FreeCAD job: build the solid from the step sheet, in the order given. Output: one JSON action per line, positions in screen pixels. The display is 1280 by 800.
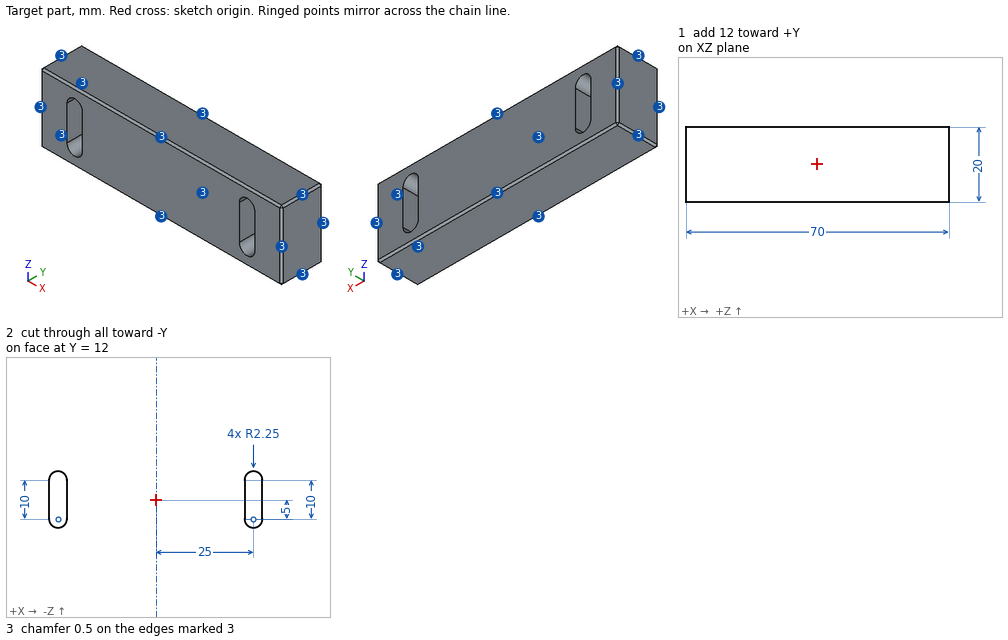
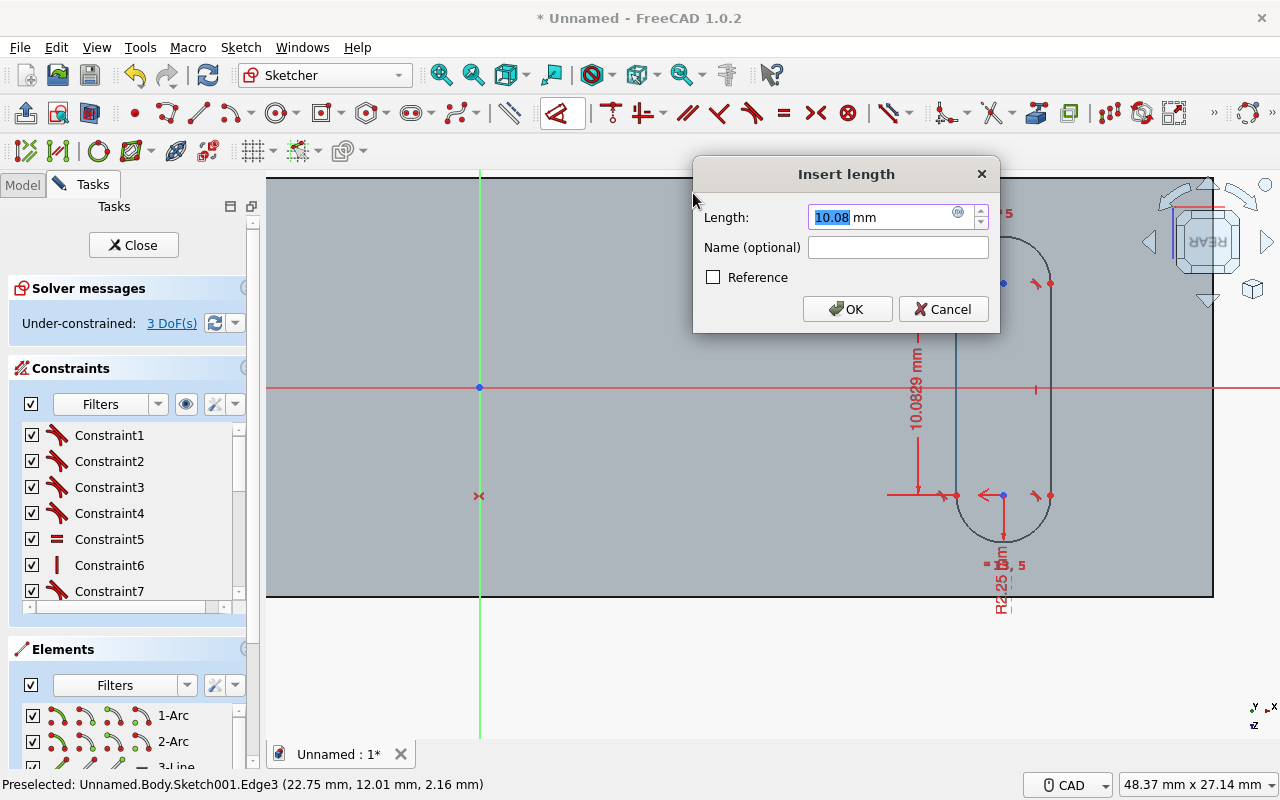
{"action": "type", "text": "10"}
{"action": "key", "text": "Return"}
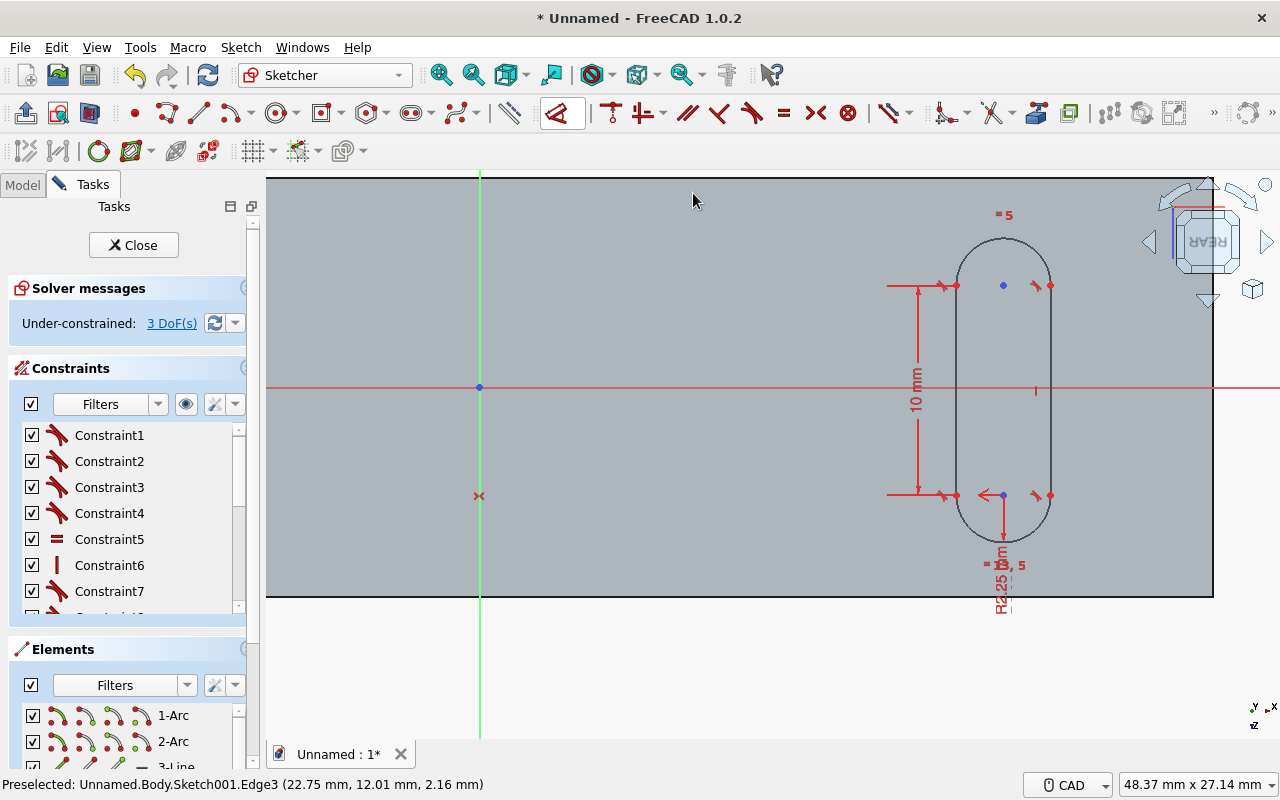
{"action": "scroll", "coordinate": [978, 536], "scroll_direction": "down", "scroll_amount": 3}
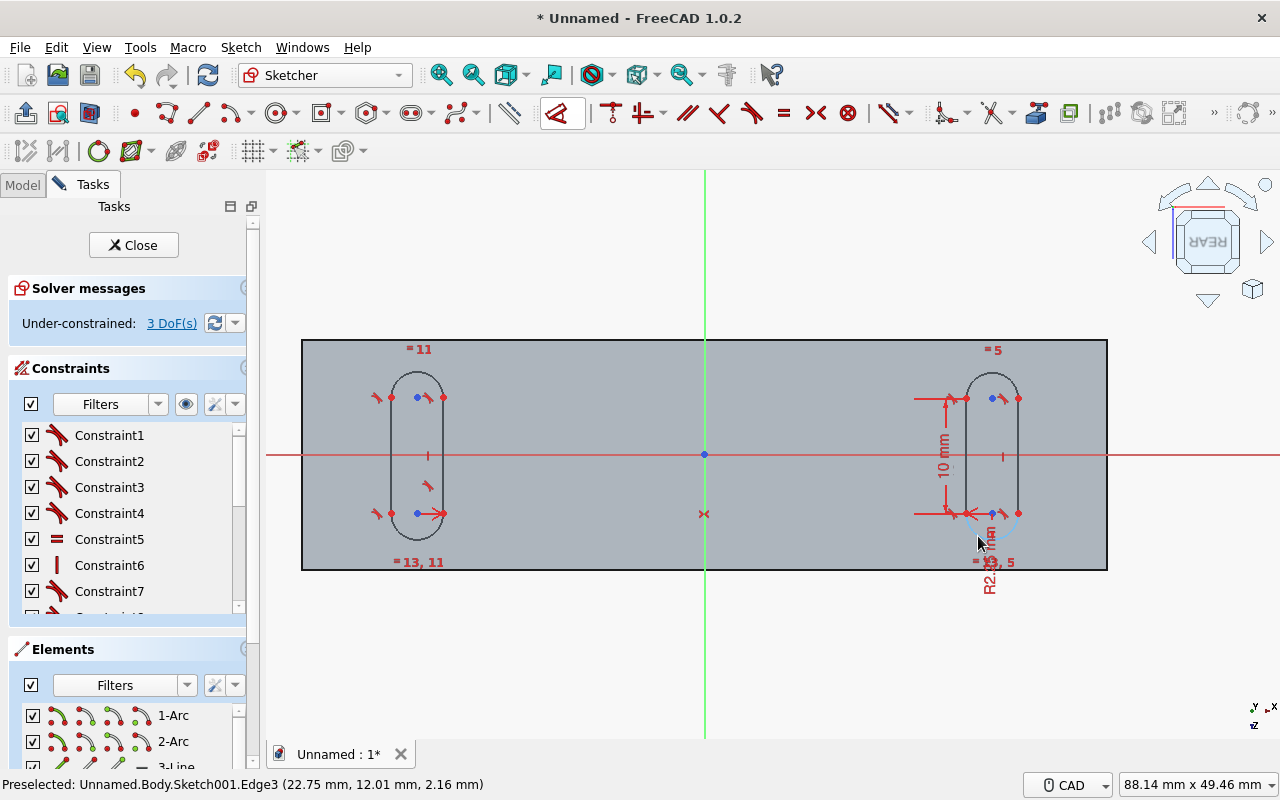
{"action": "left_click", "coordinate": [391, 479]}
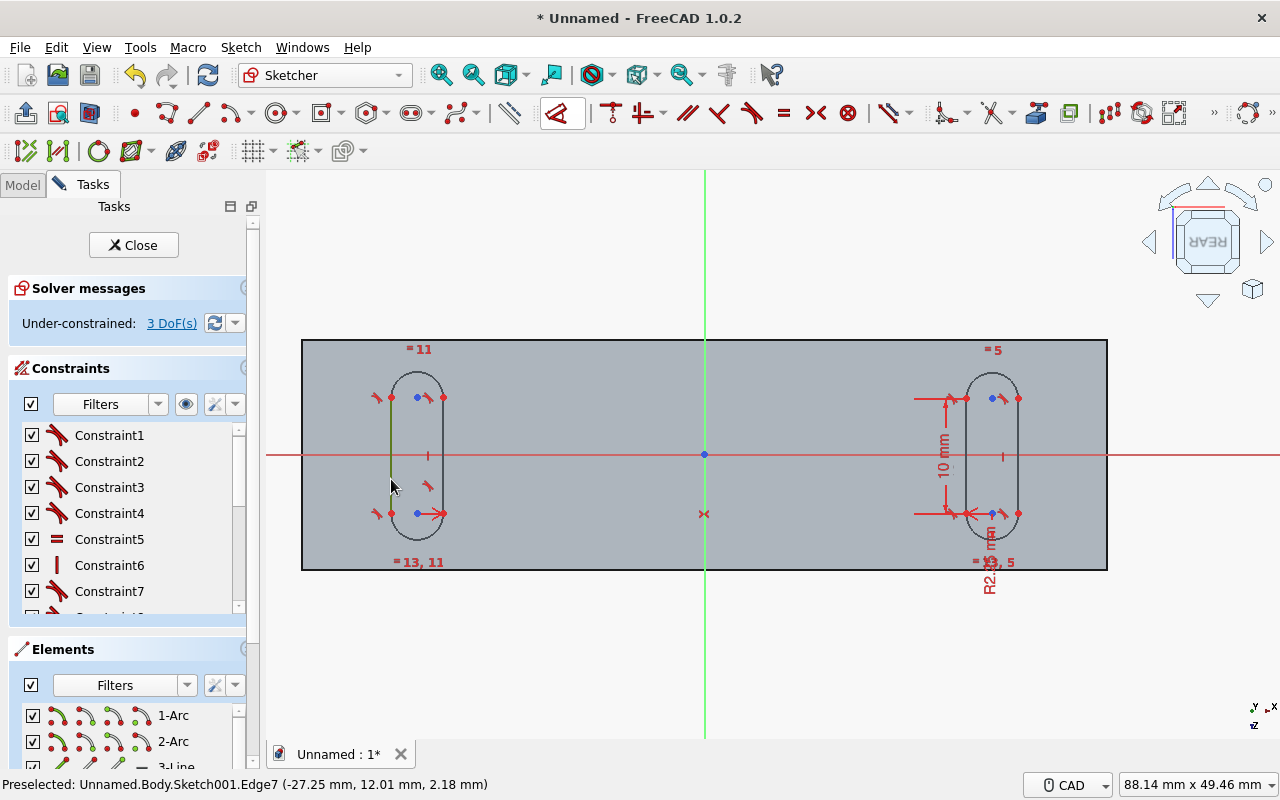
{"action": "key", "text": "i"}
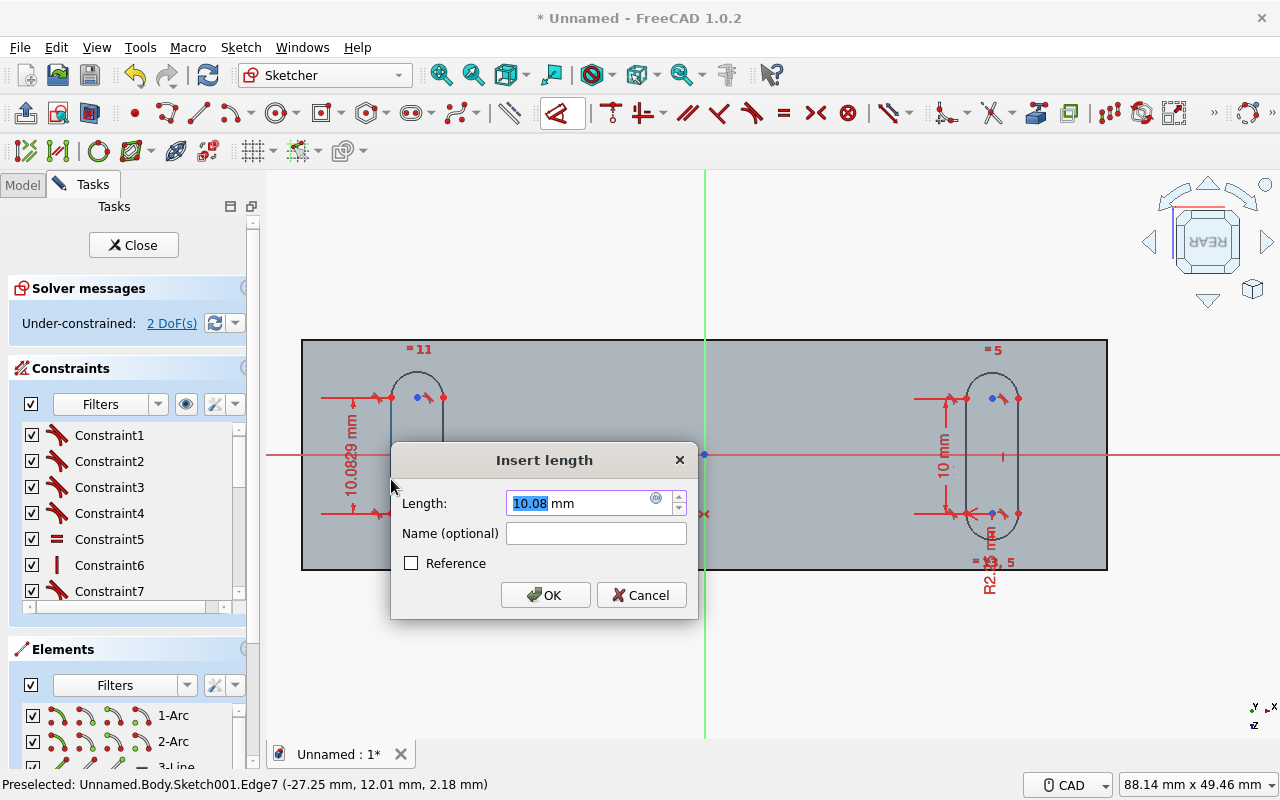
{"action": "type", "text": "10"}
{"action": "key", "text": "Return"}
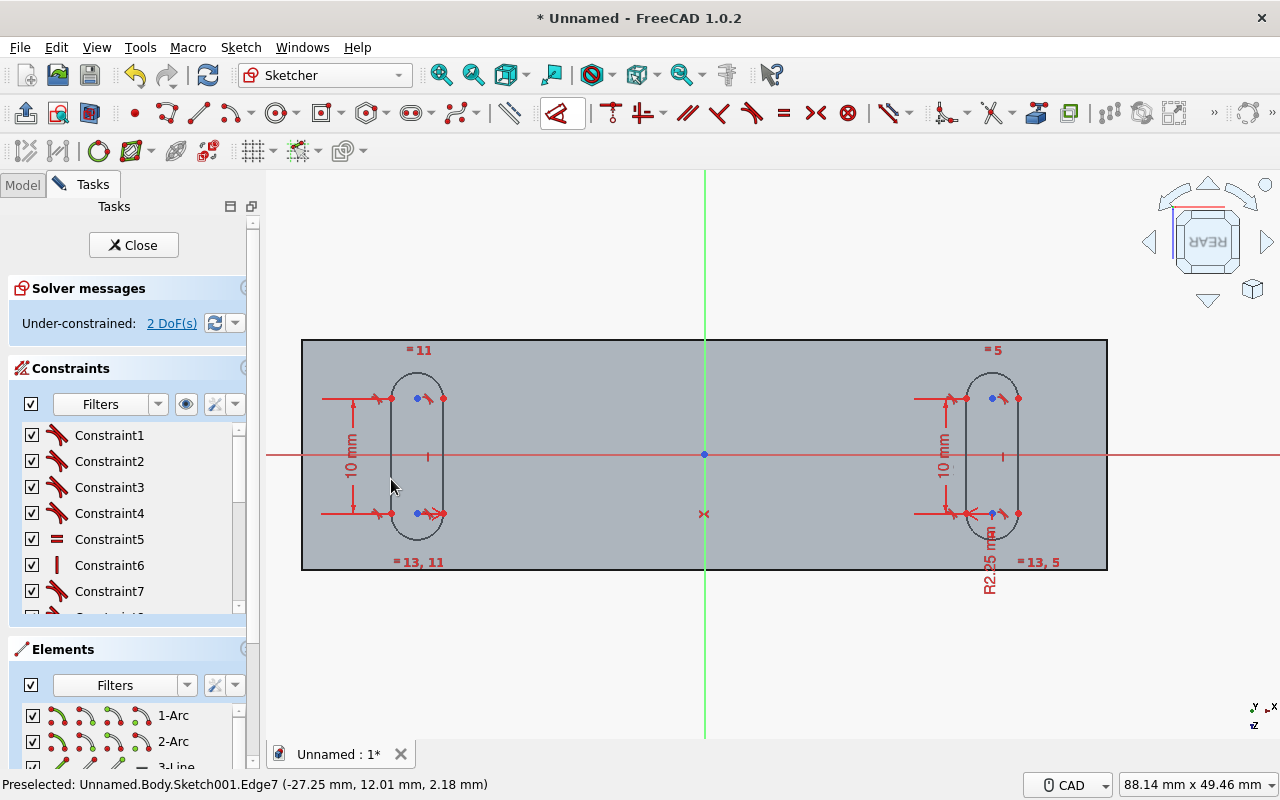
{"action": "left_click", "coordinate": [966, 514]}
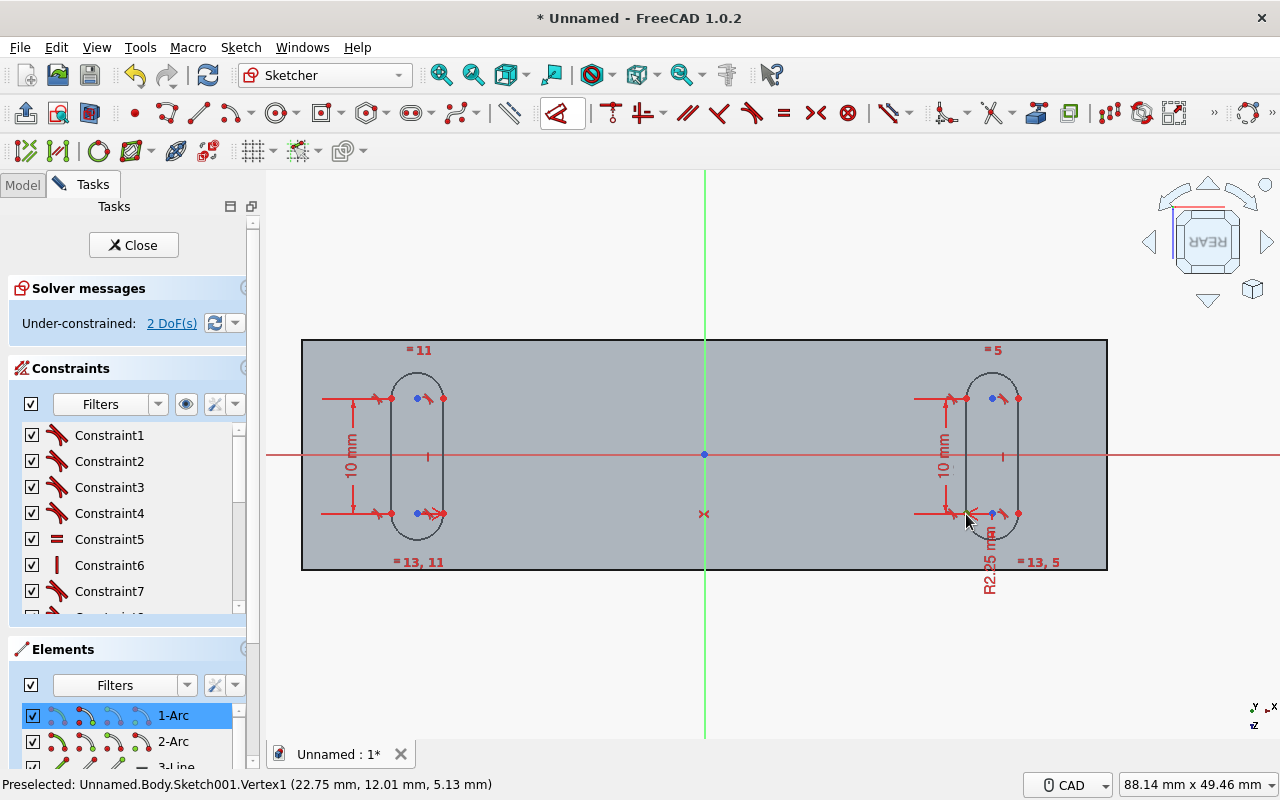
{"action": "key", "text": "i"}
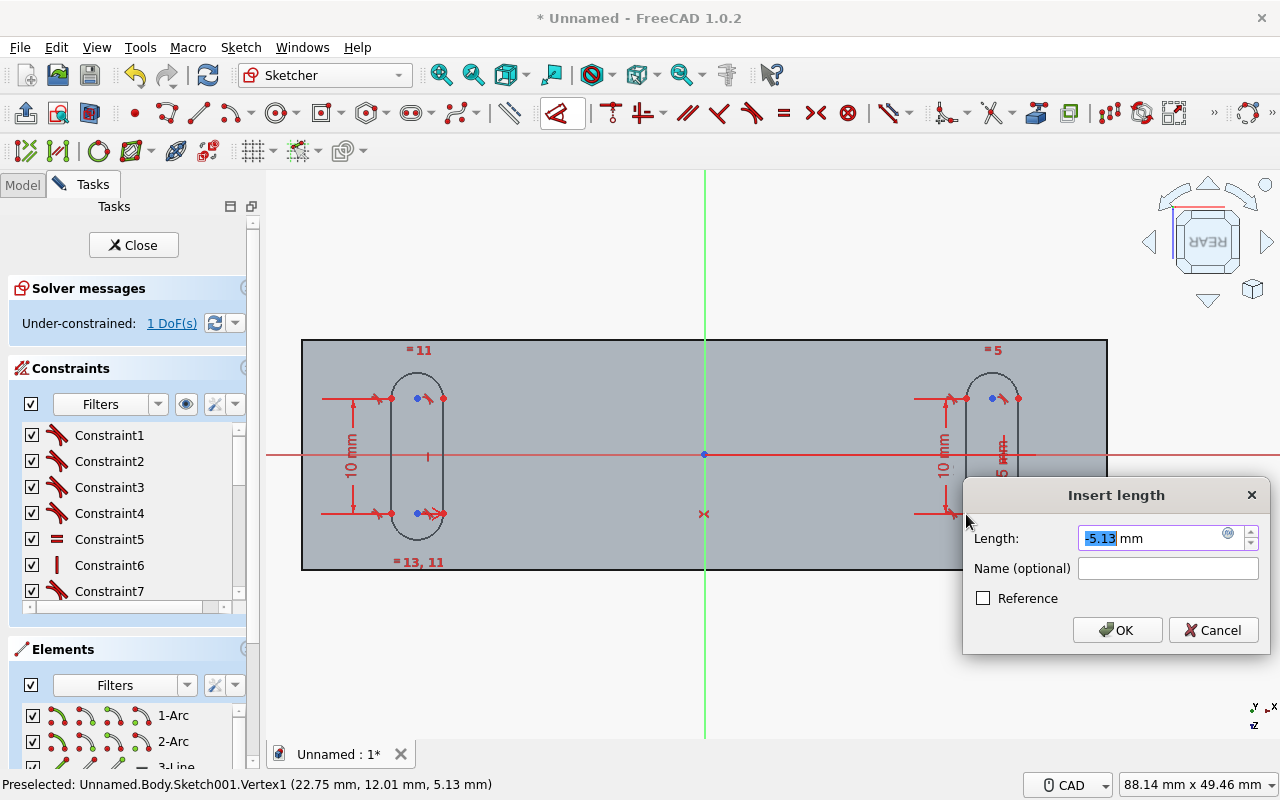
{"action": "type", "text": "-5"}
{"action": "key", "text": "Return"}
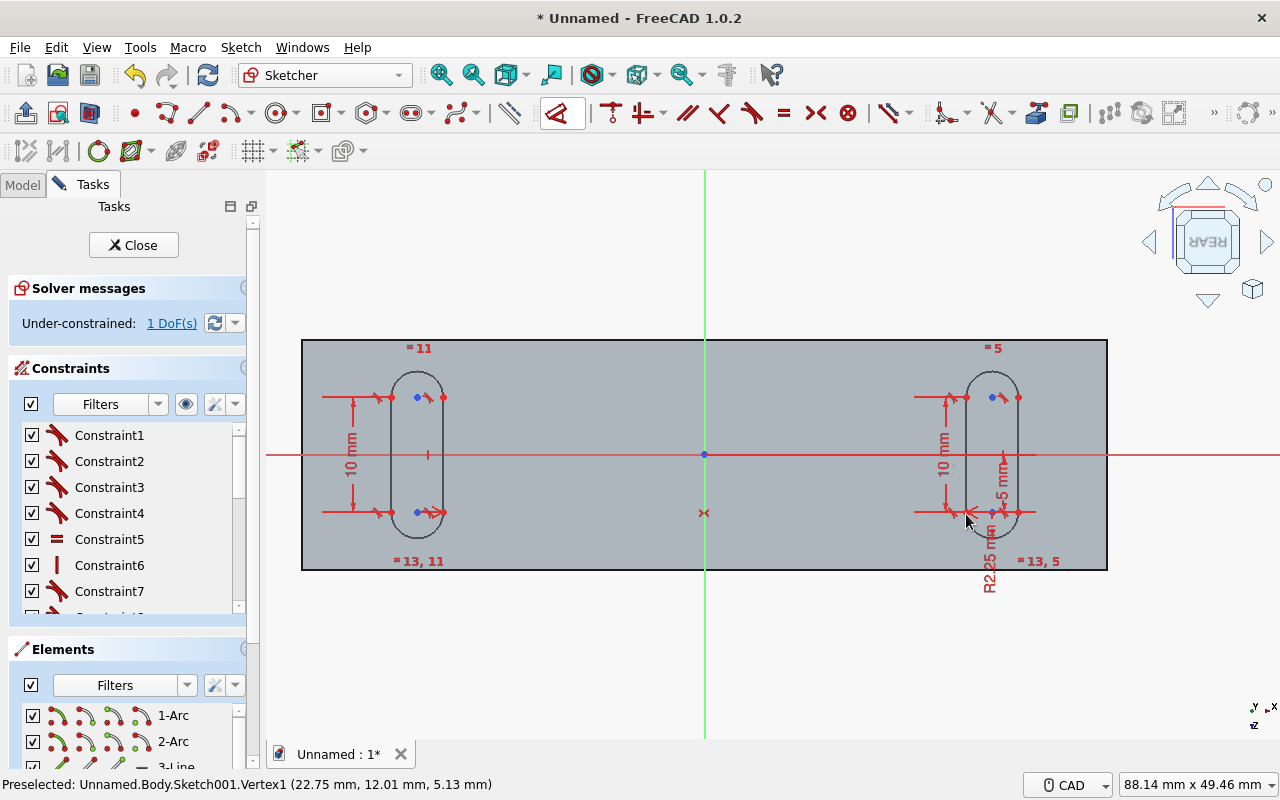
{"action": "left_click", "coordinate": [992, 512]}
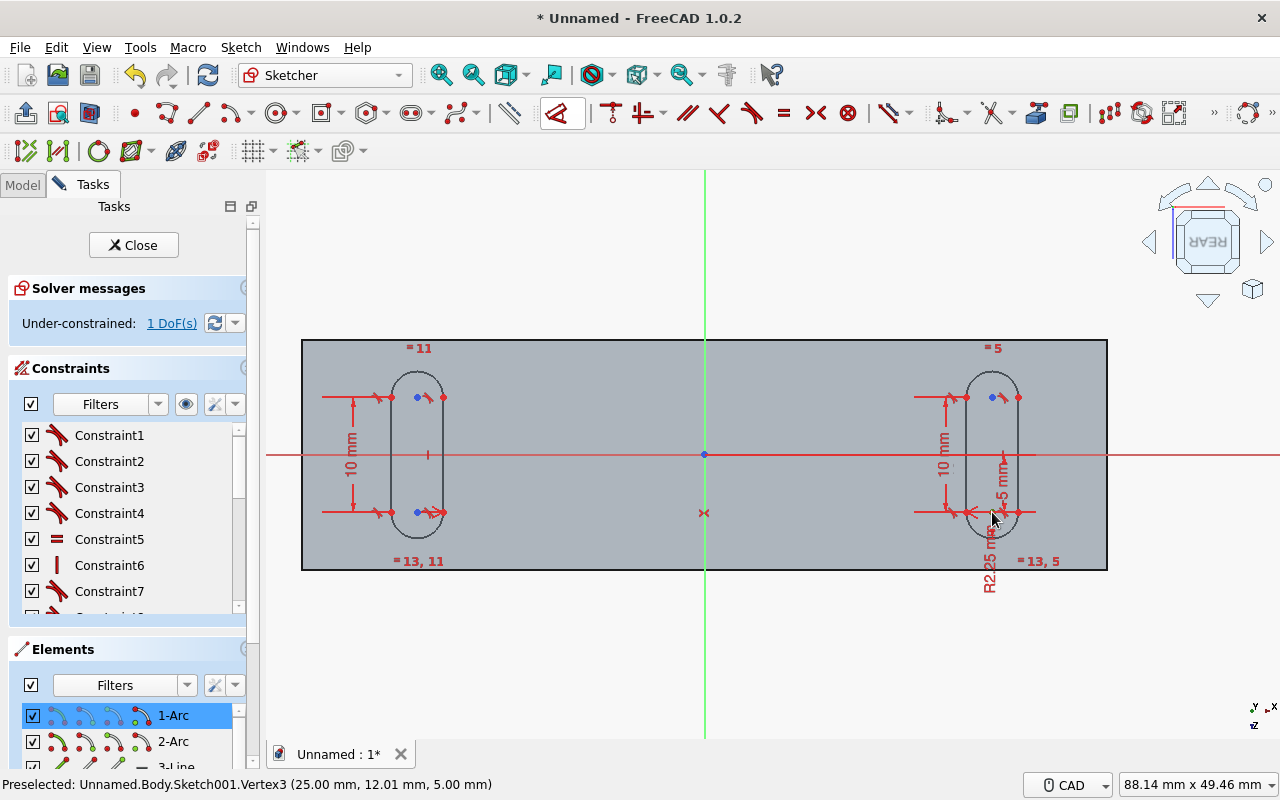
{"action": "key", "text": "l"}